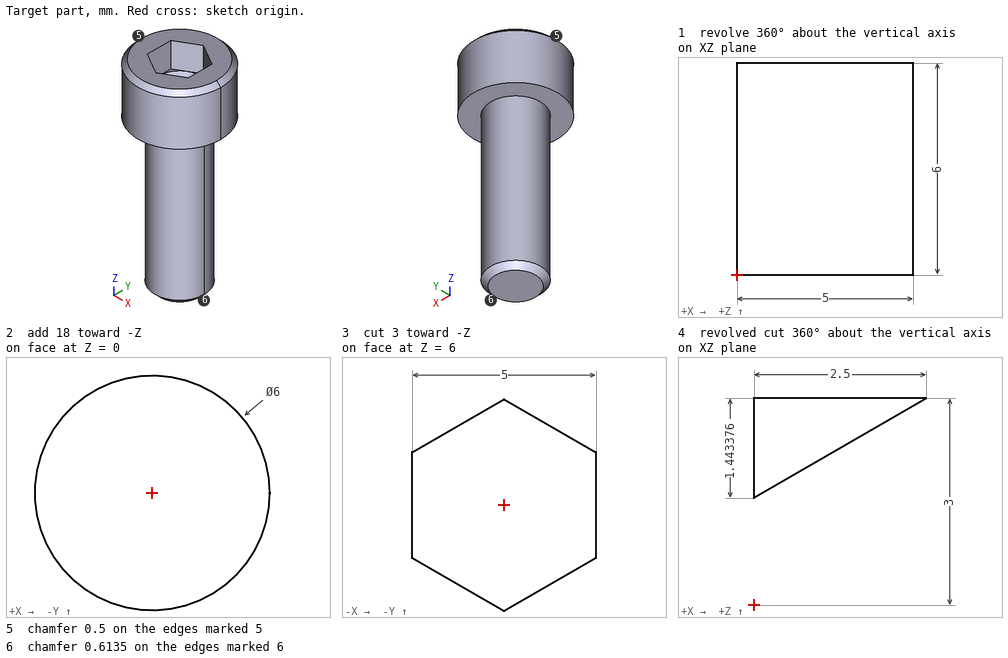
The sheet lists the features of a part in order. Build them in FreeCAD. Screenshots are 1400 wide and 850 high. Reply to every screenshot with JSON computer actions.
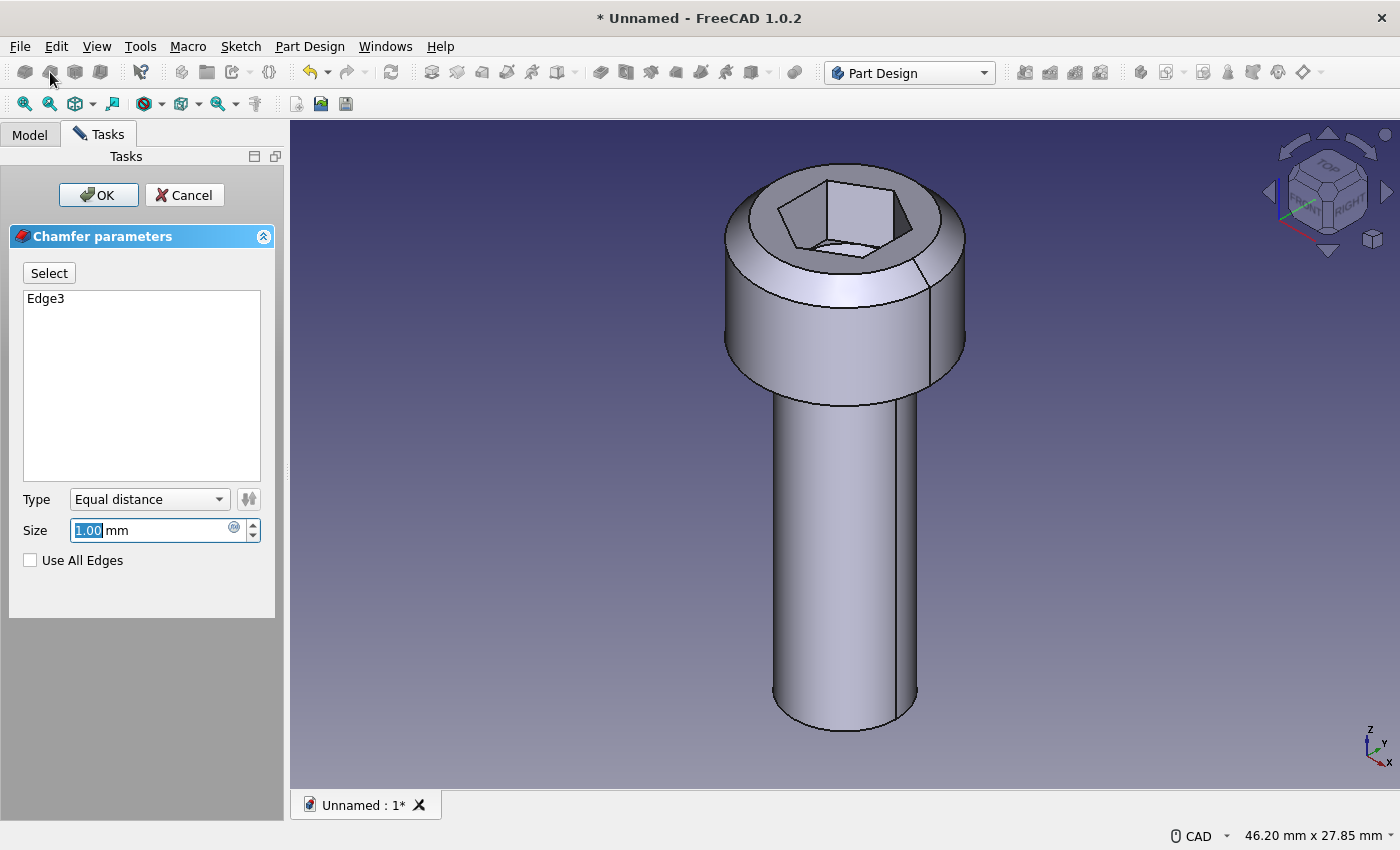
{"action": "type", "text": "0.5"}
{"action": "key", "text": "Tab"}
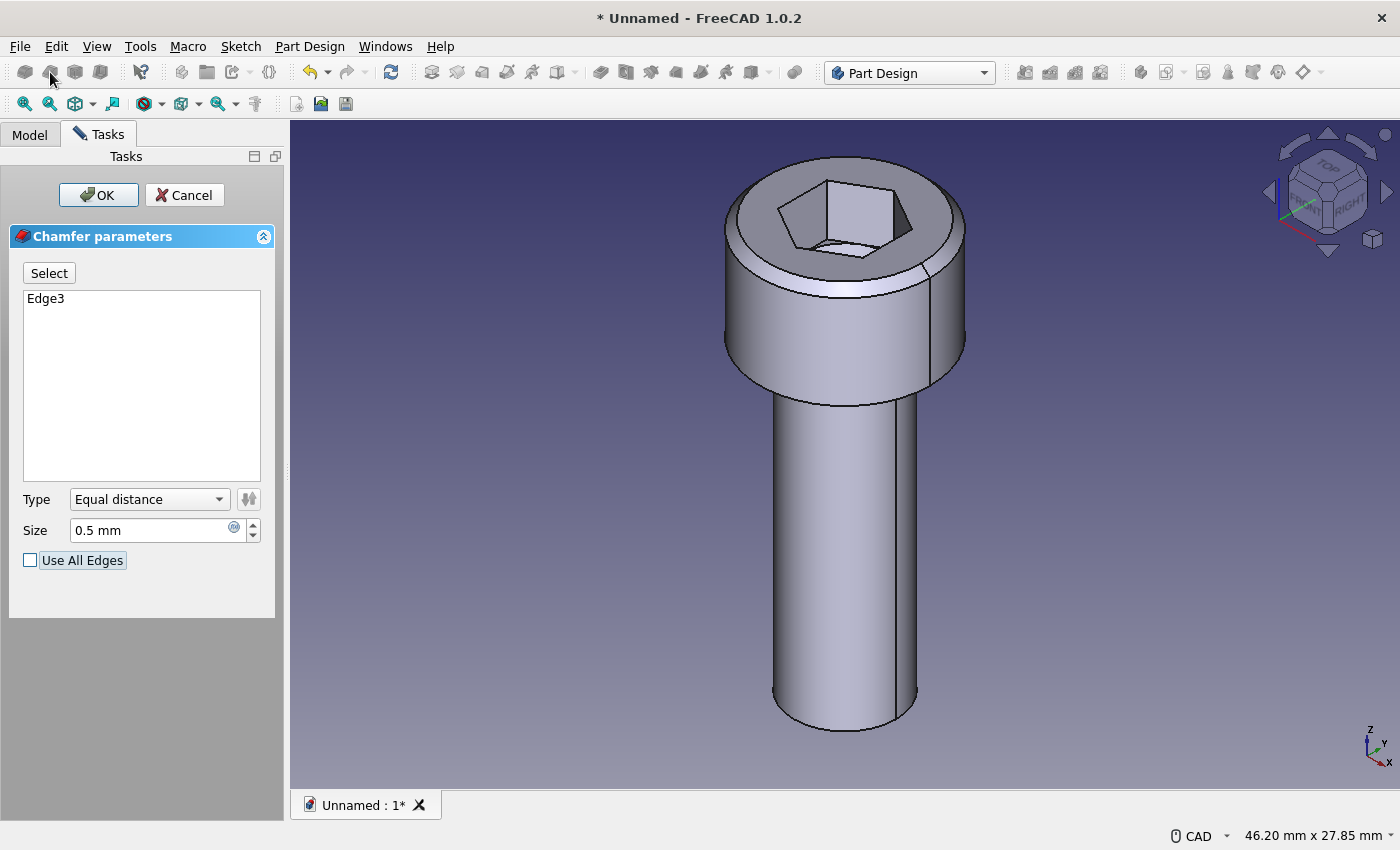
{"action": "left_click", "coordinate": [99, 195]}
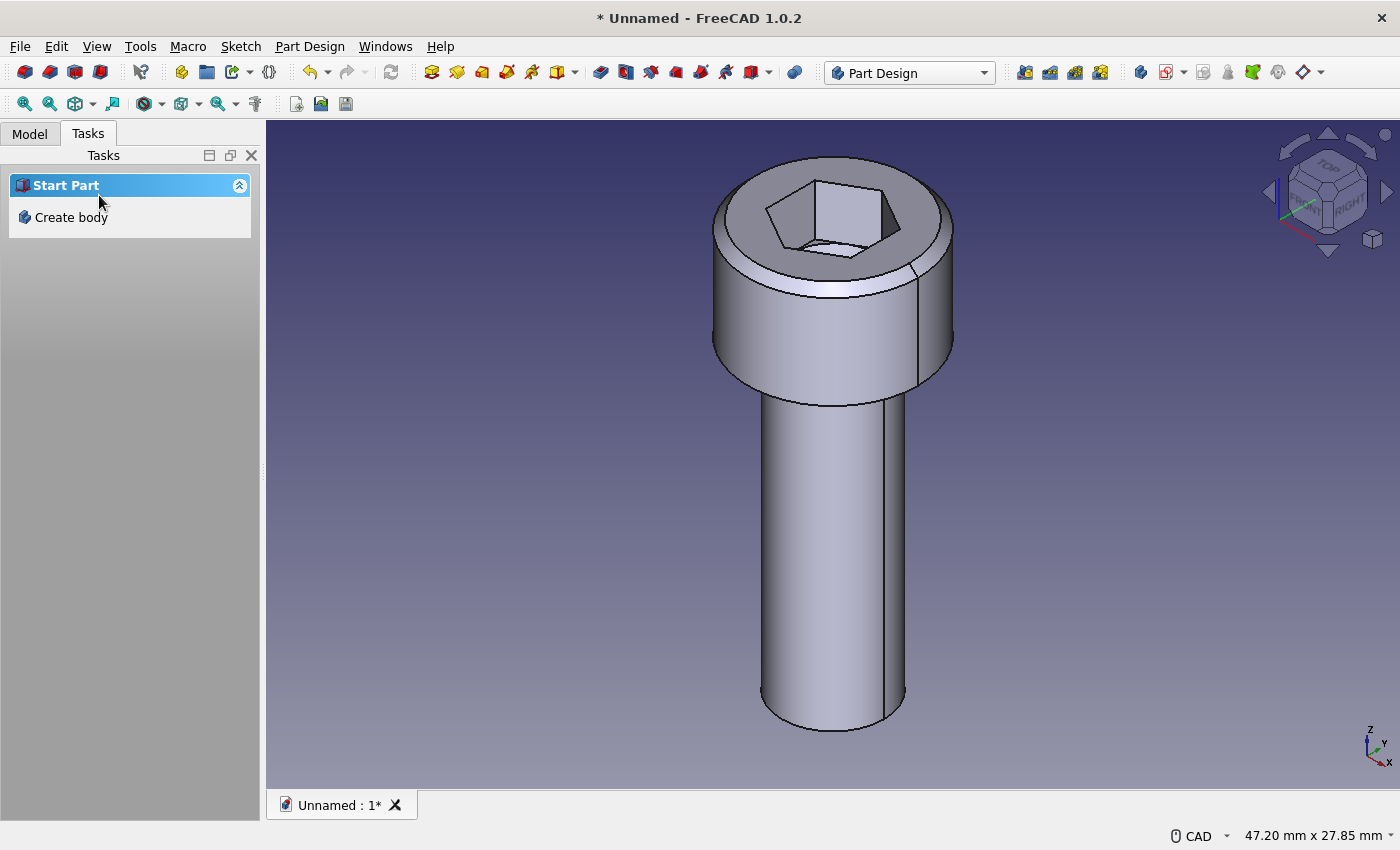
{"action": "key", "text": "2"}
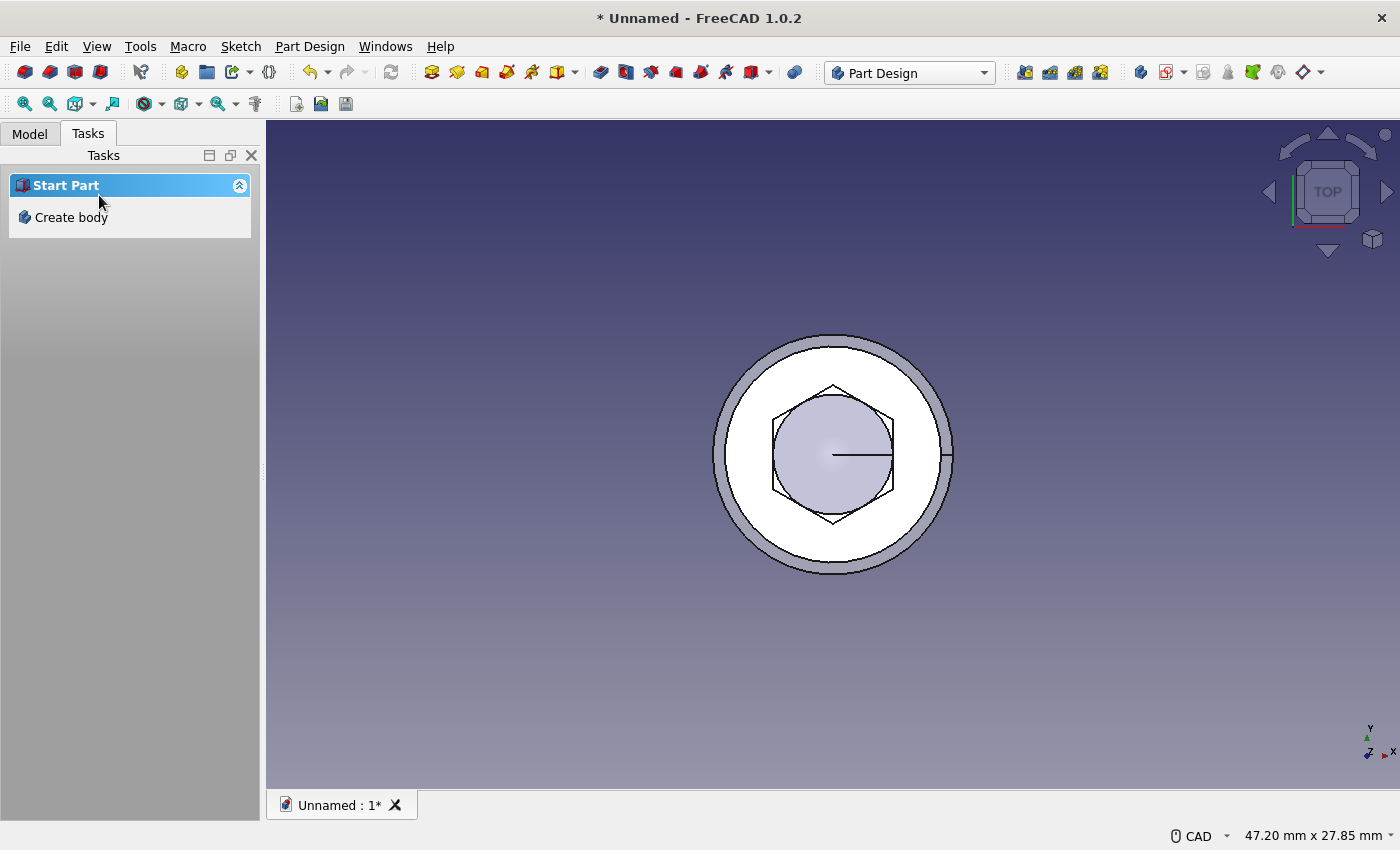
{"action": "left_click", "coordinate": [25, 104]}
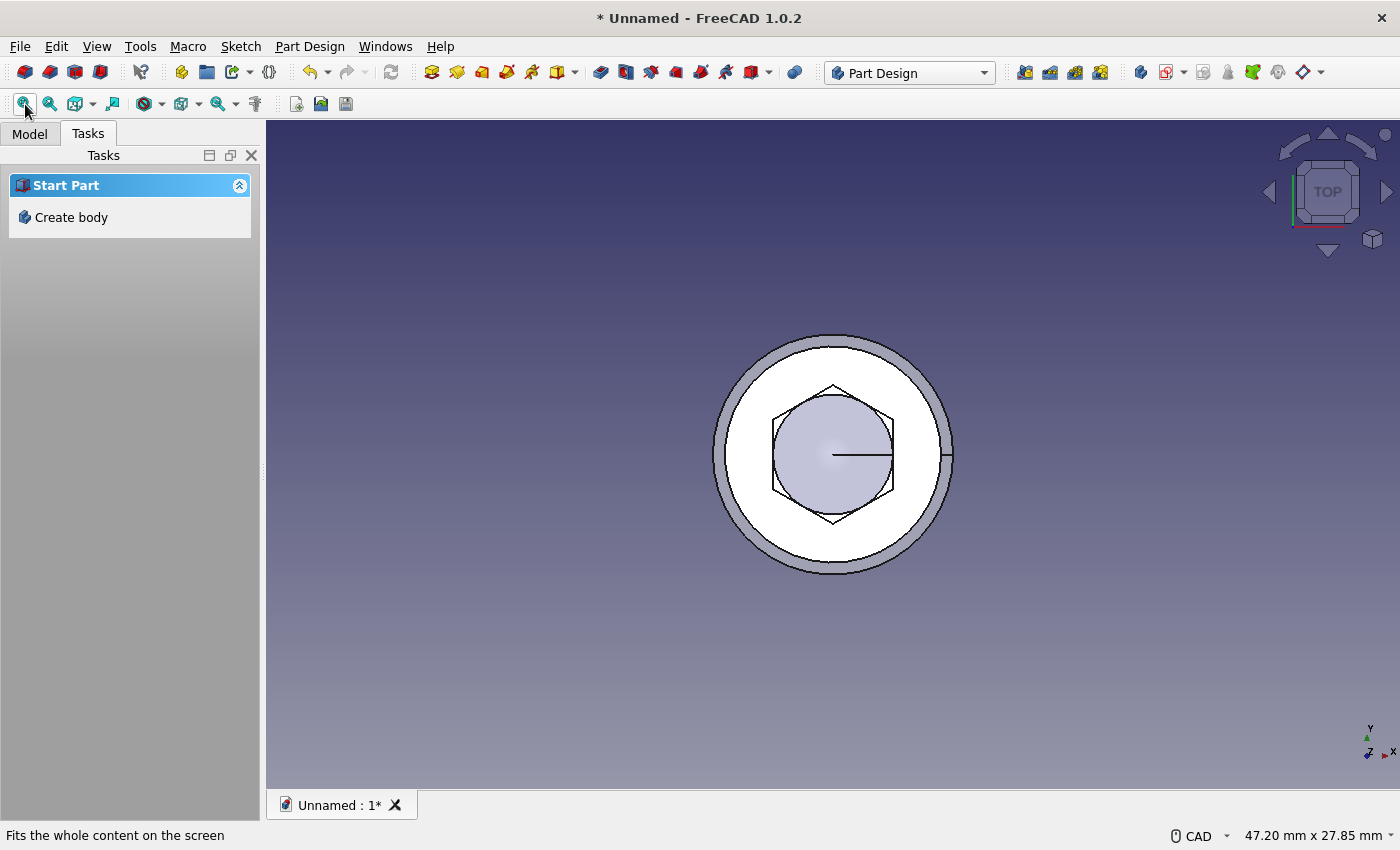
{"action": "key", "text": "0"}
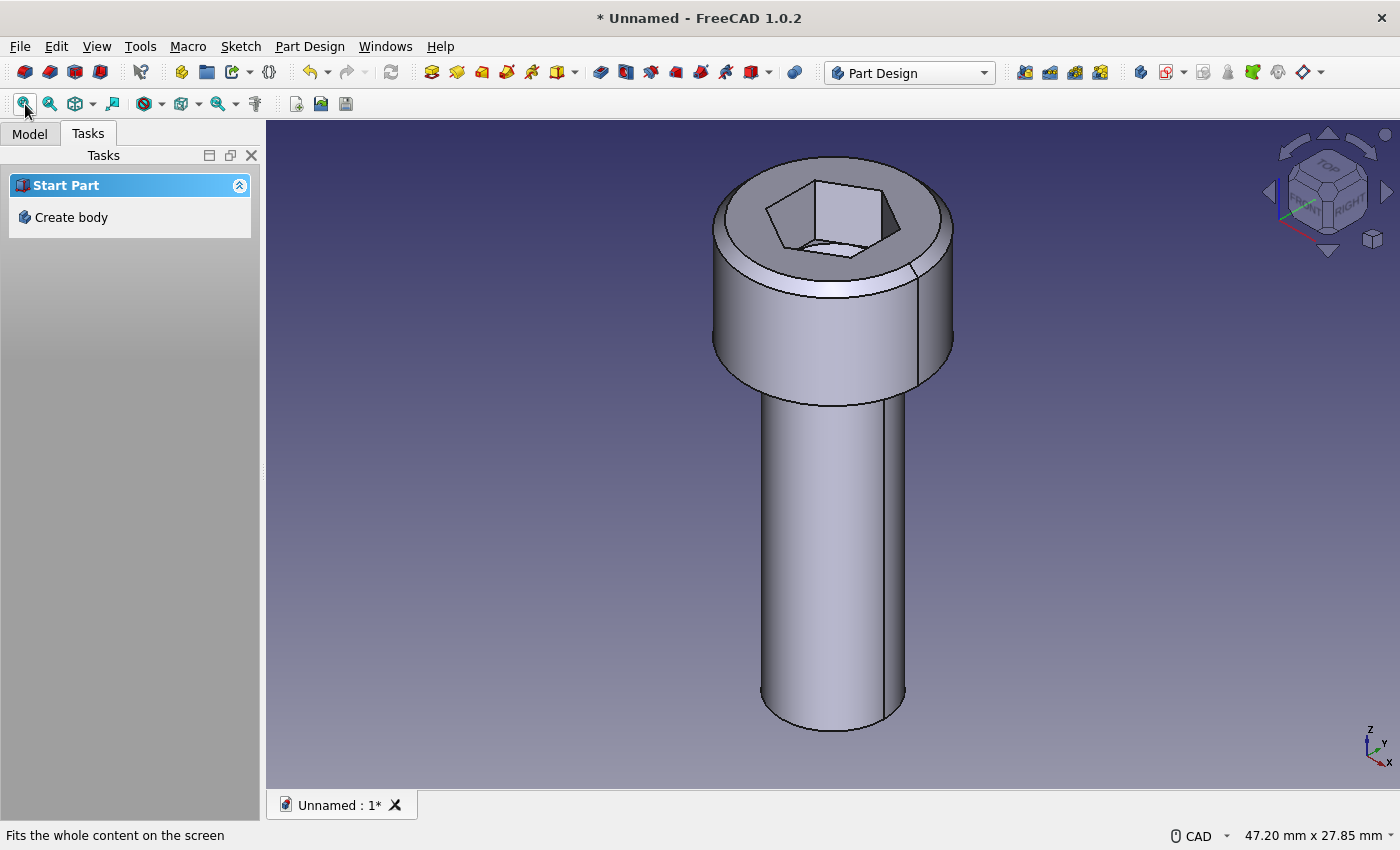
{"action": "key", "text": "1"}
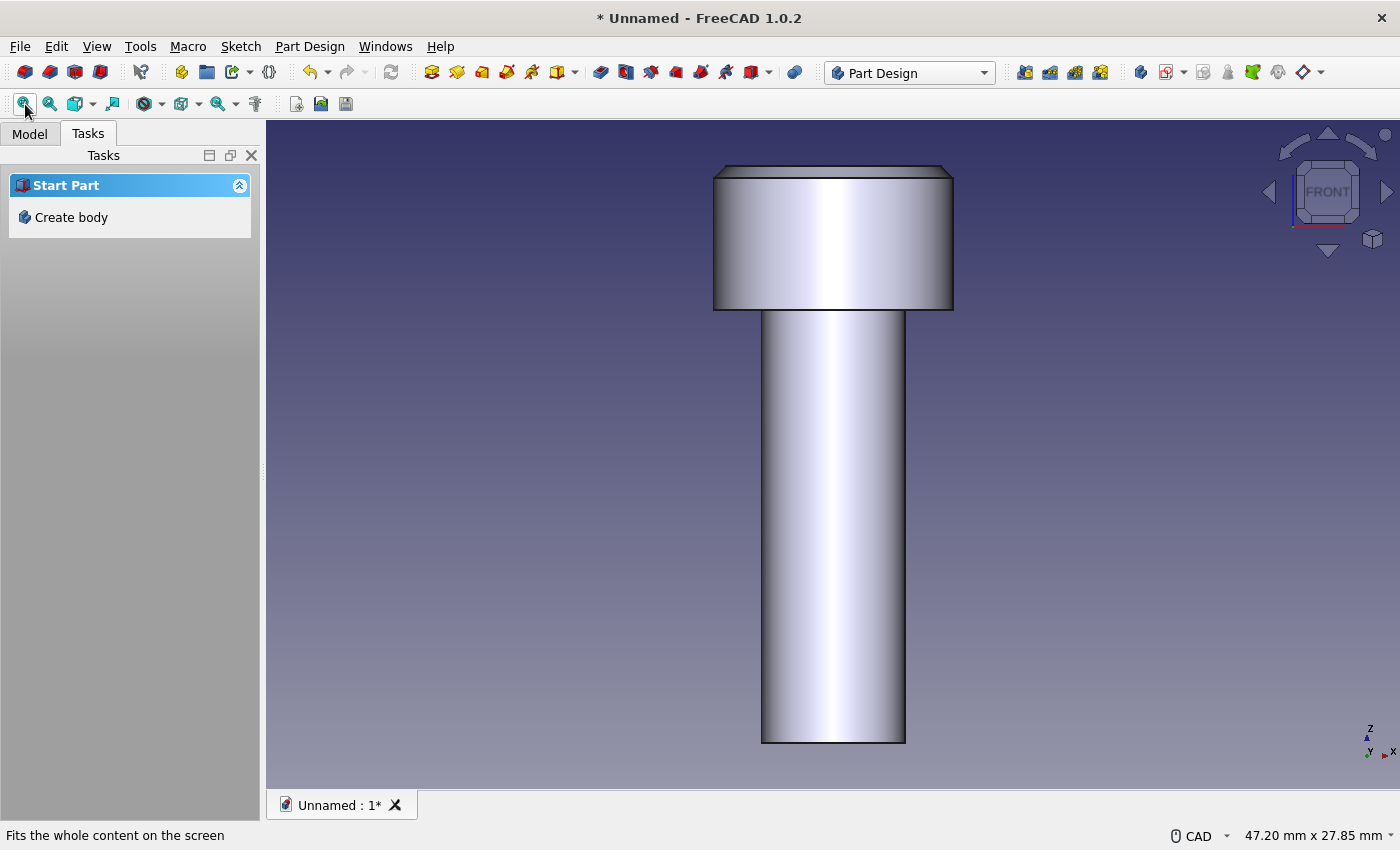
{"action": "left_click", "coordinate": [886, 742]}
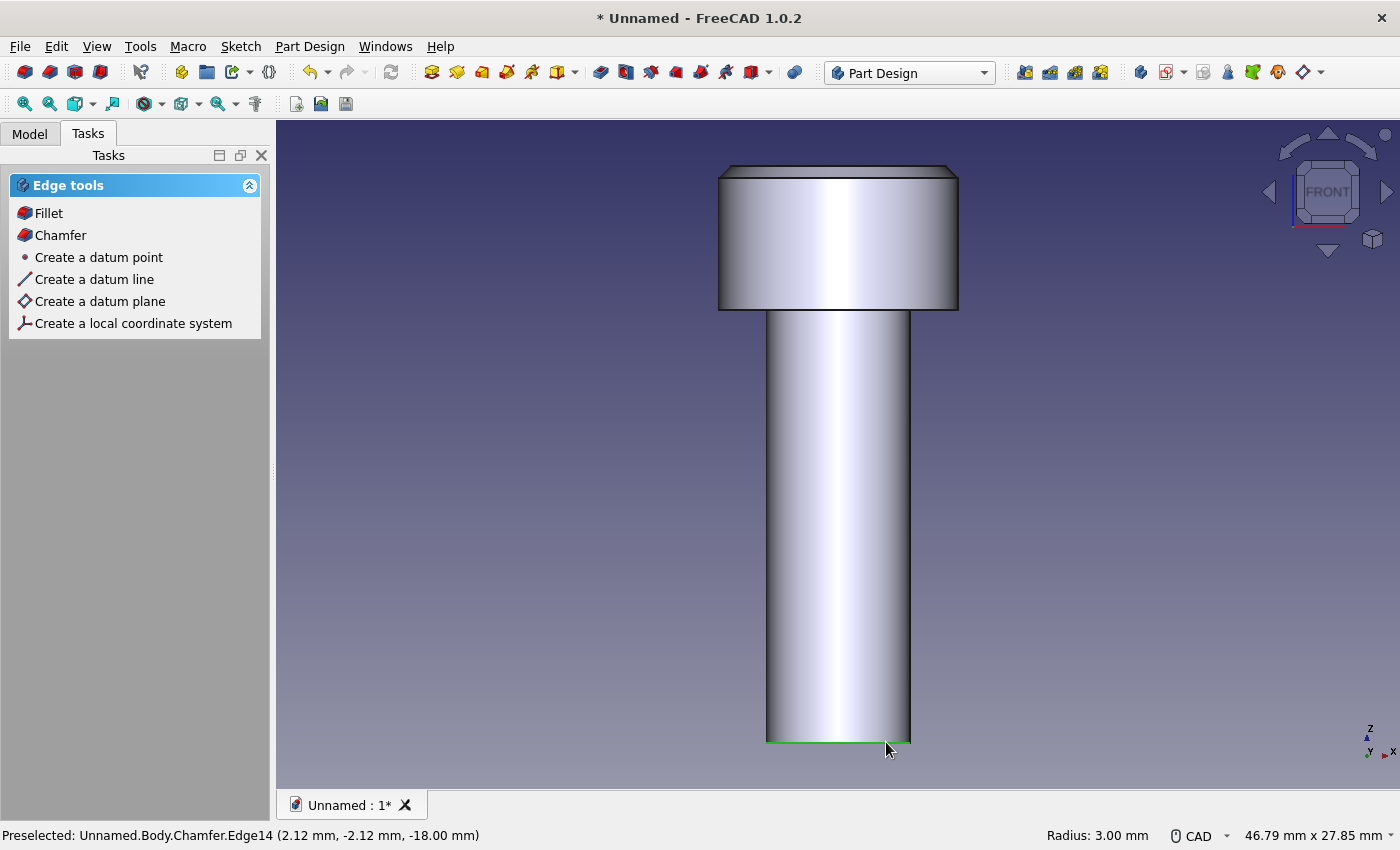
{"action": "left_click", "coordinate": [50, 72]}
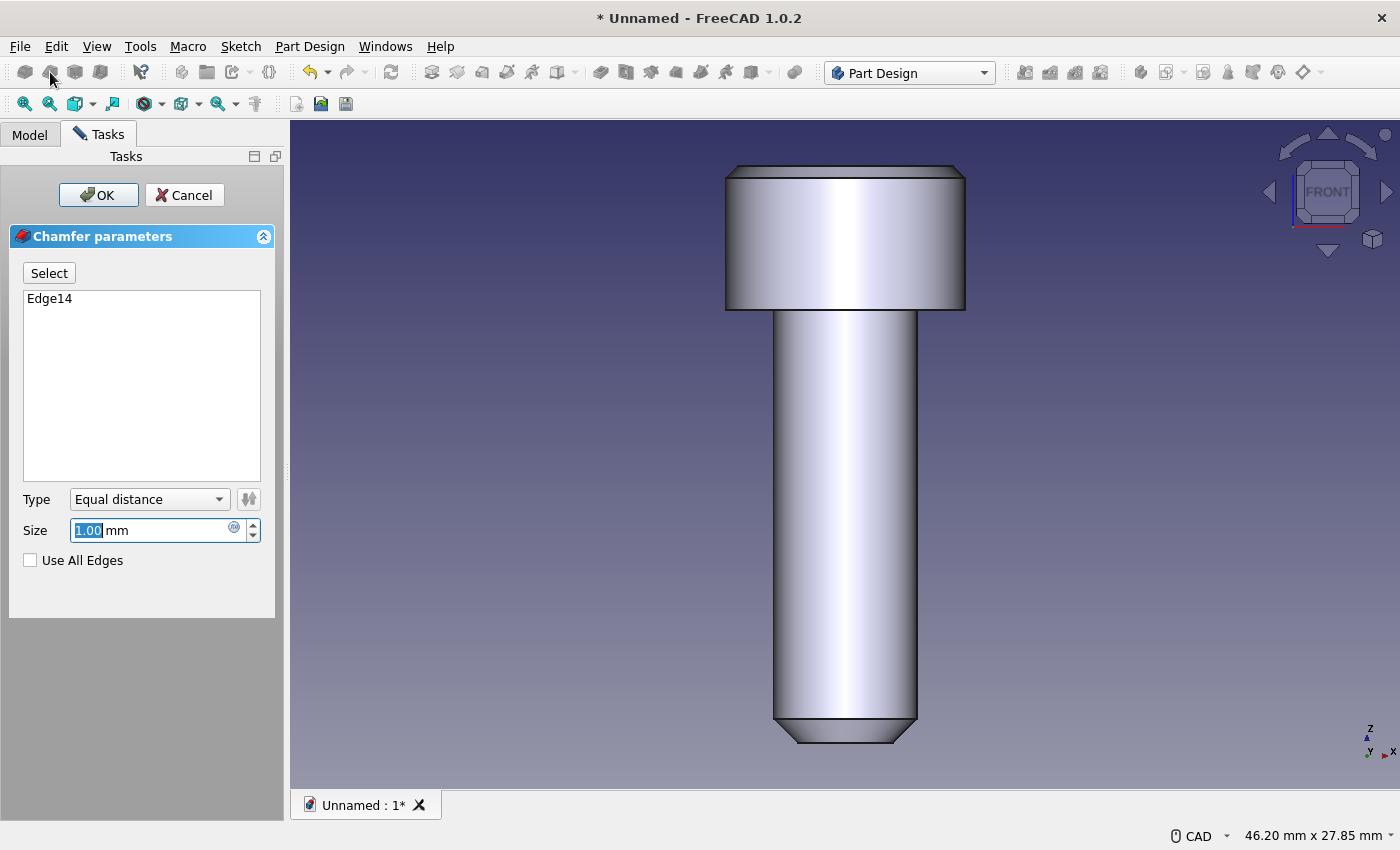
{"action": "type", "text": "0.6135"}
{"action": "key", "text": "Tab"}